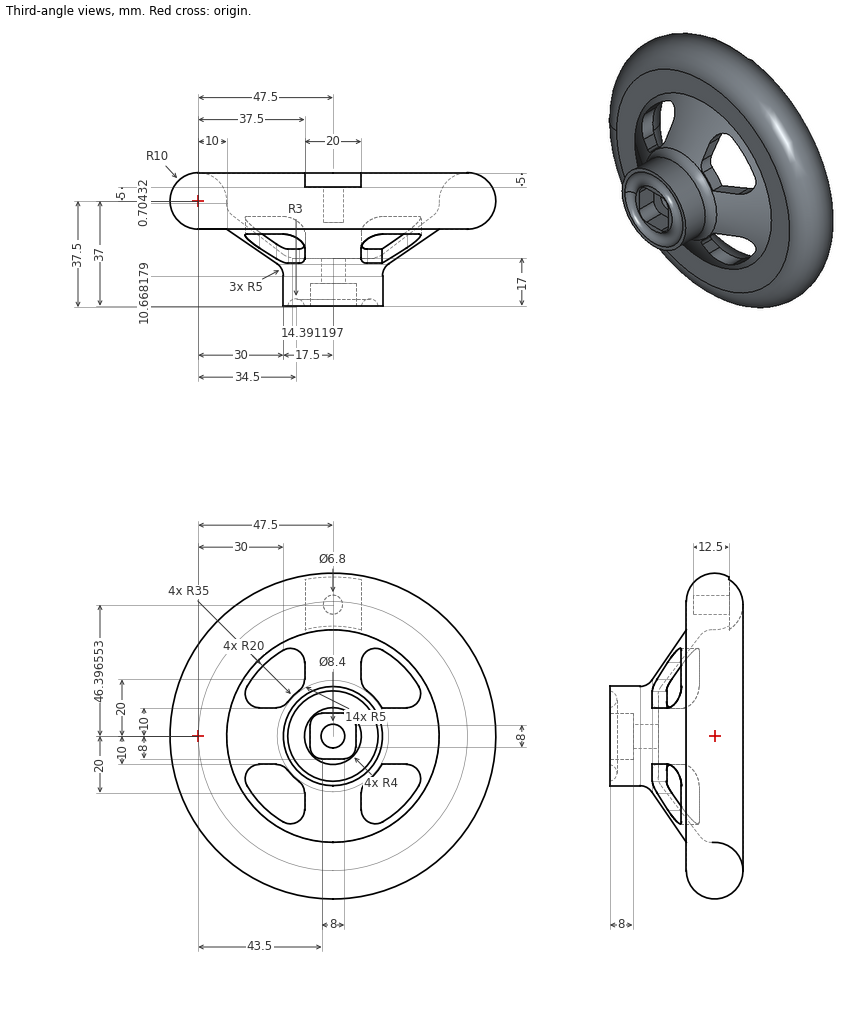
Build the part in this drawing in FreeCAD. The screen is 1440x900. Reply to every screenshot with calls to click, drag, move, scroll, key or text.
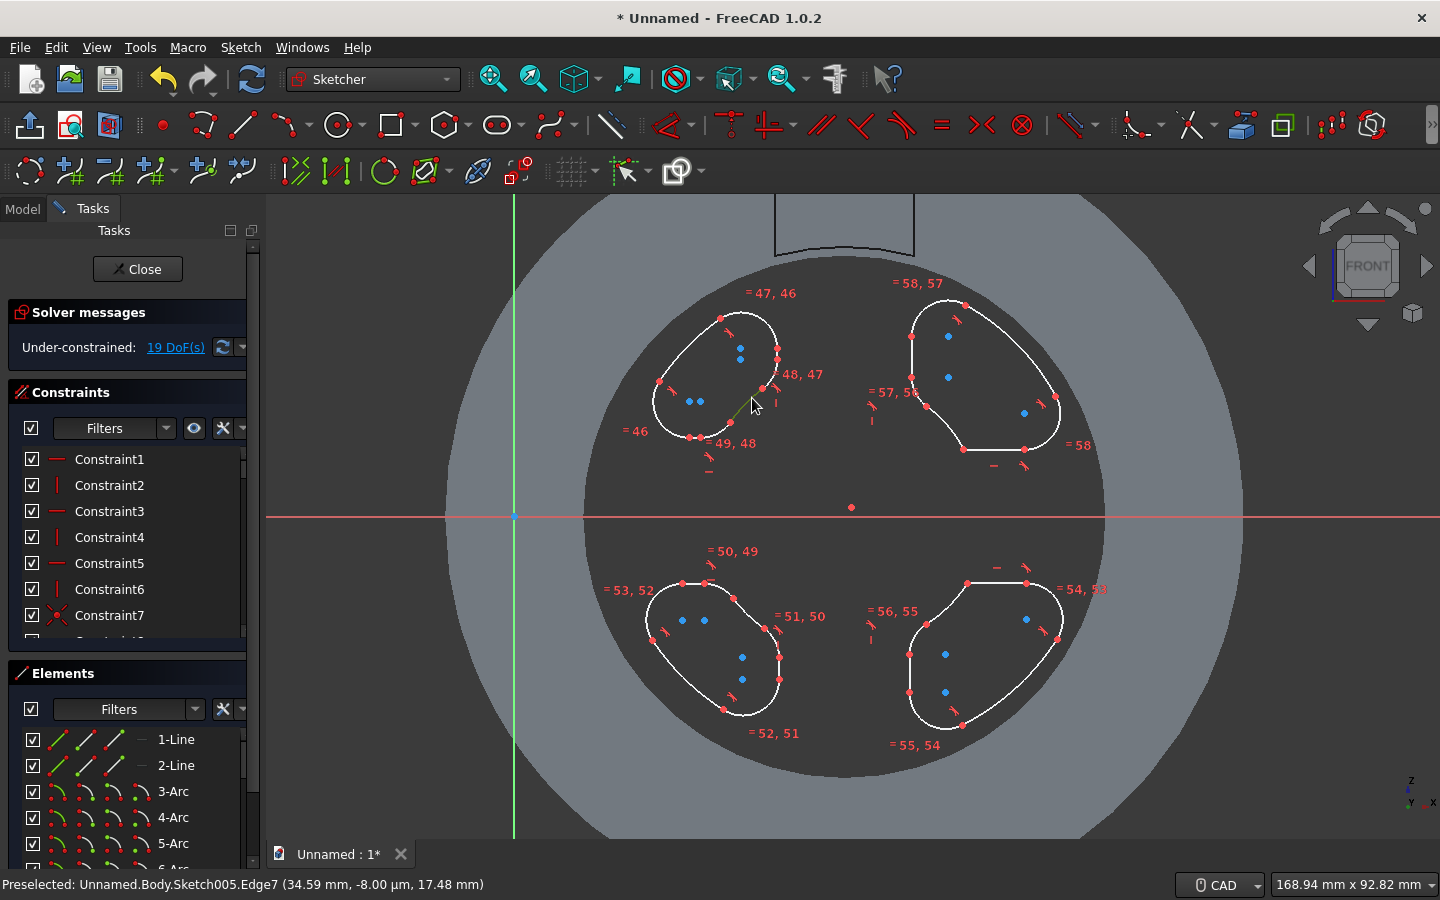
click(741, 608)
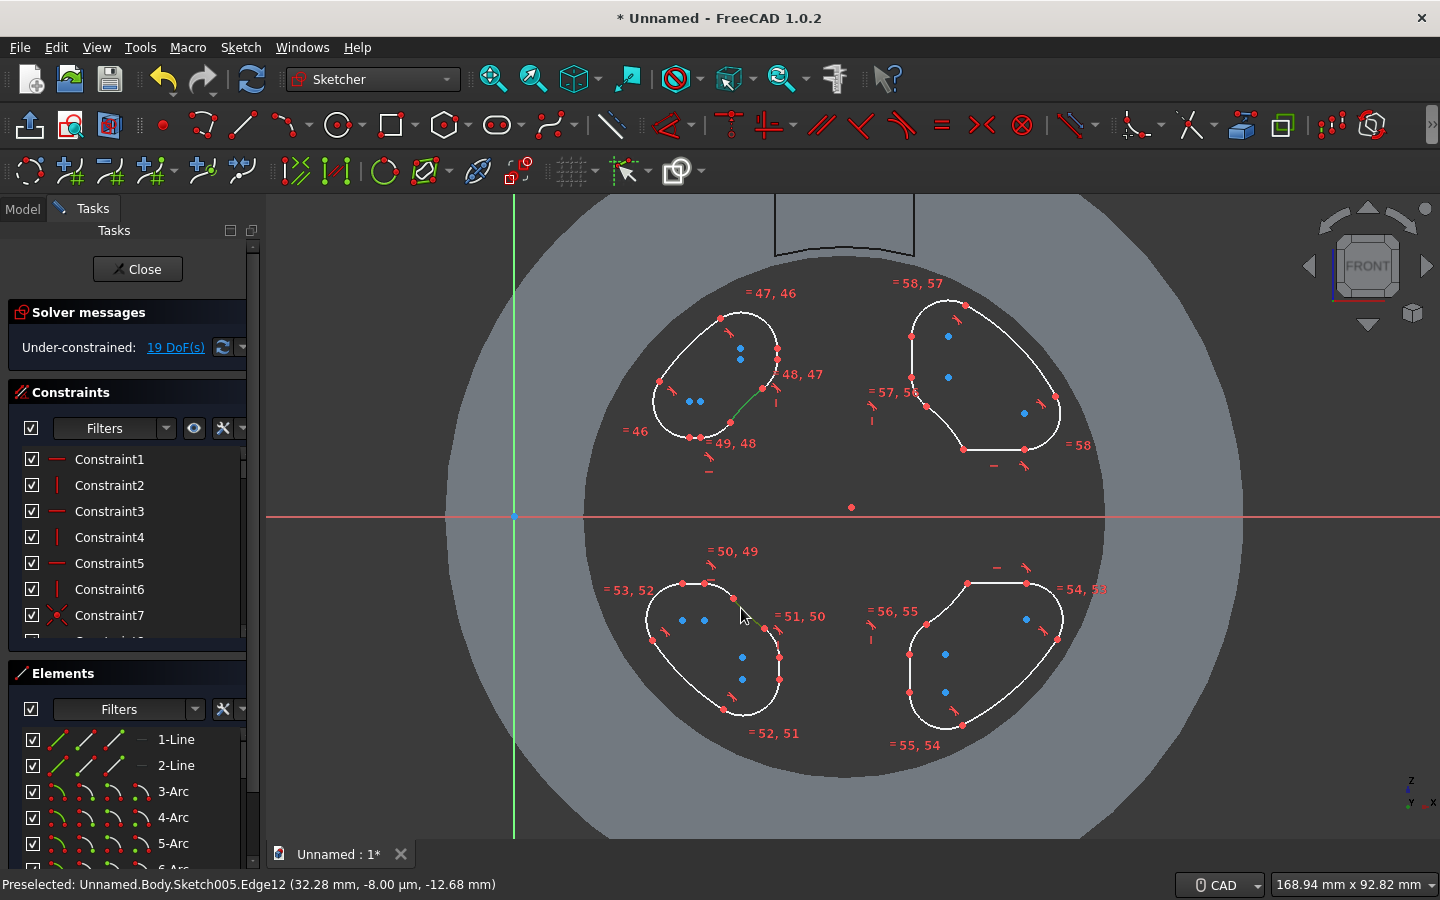
click(940, 614)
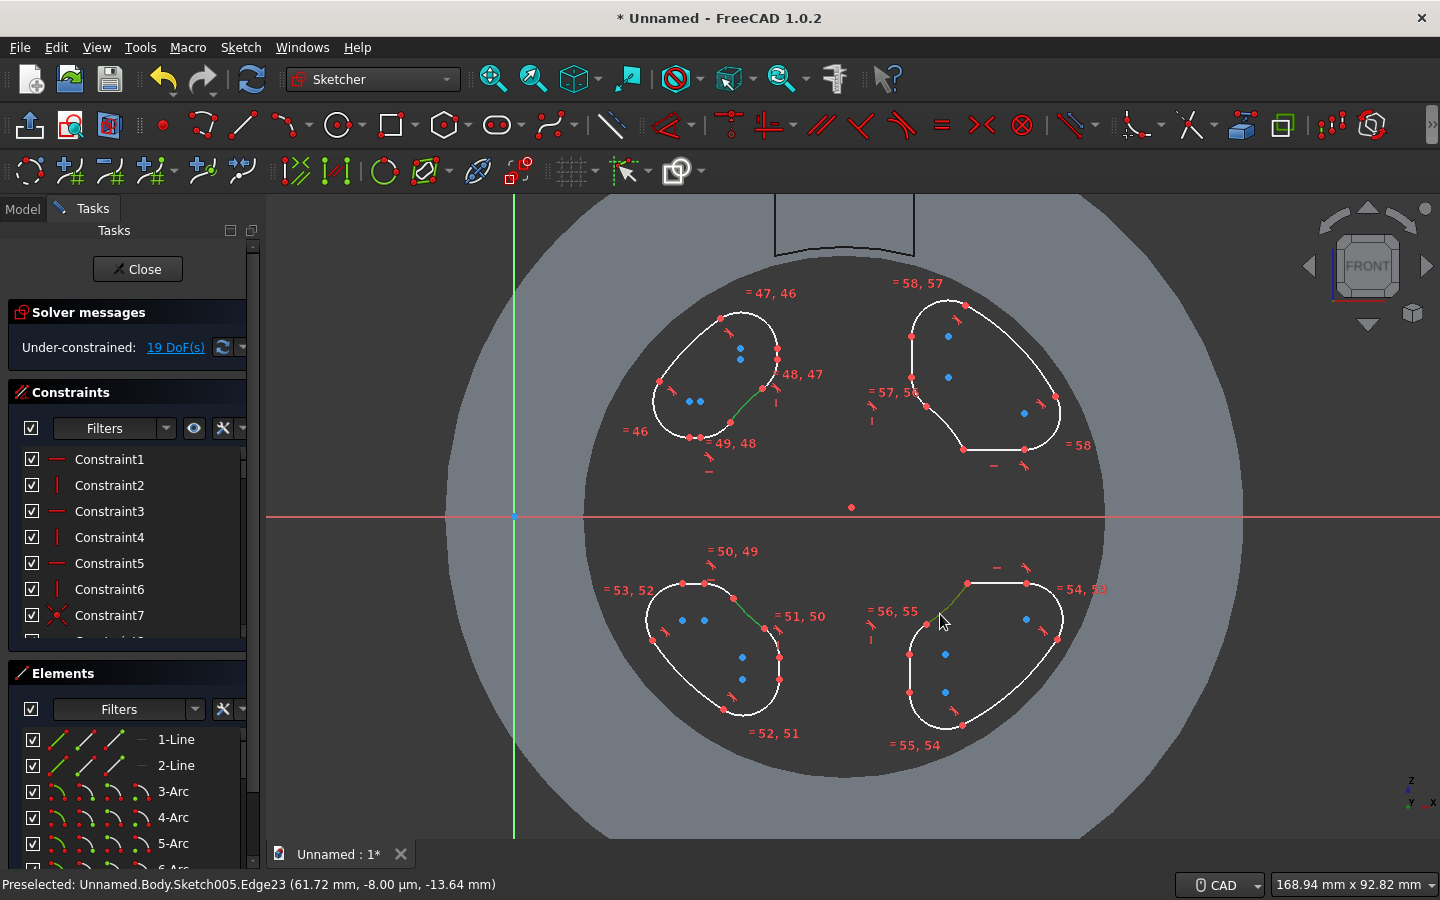
click(955, 435)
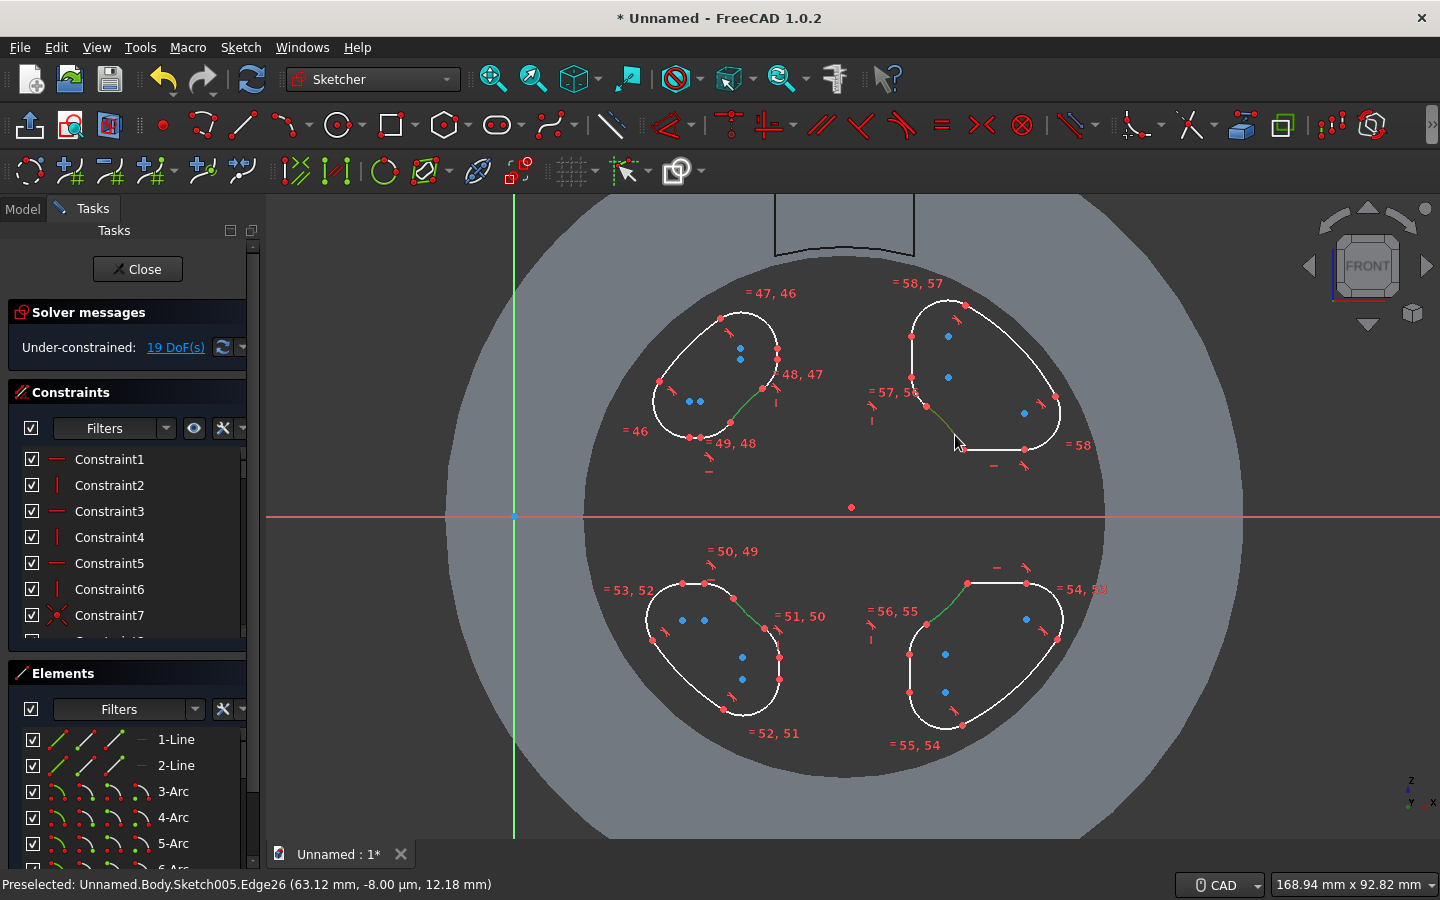
click(942, 126)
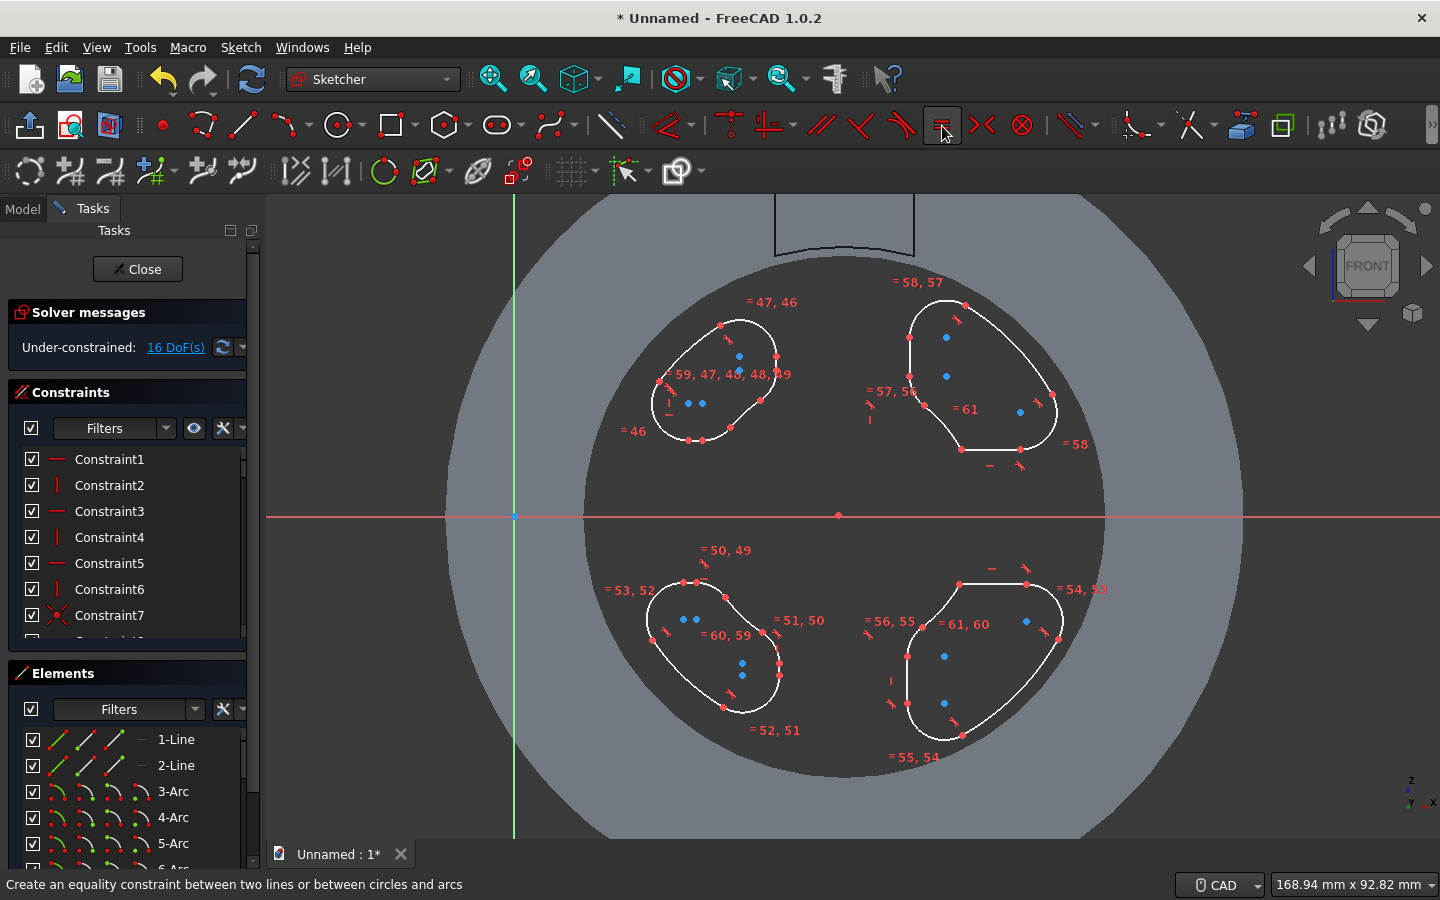
click(700, 340)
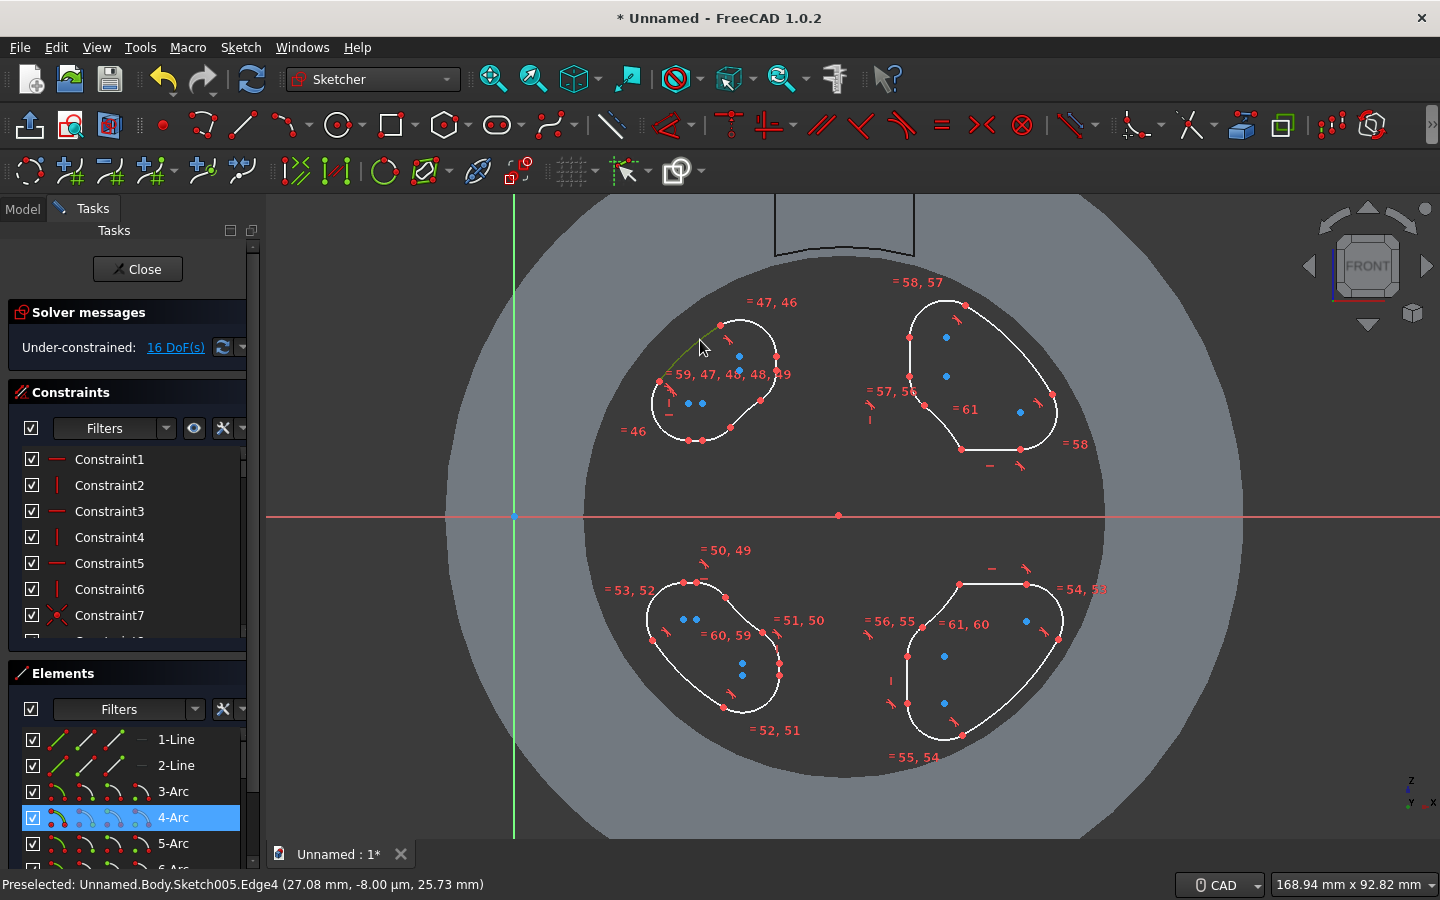
click(671, 663)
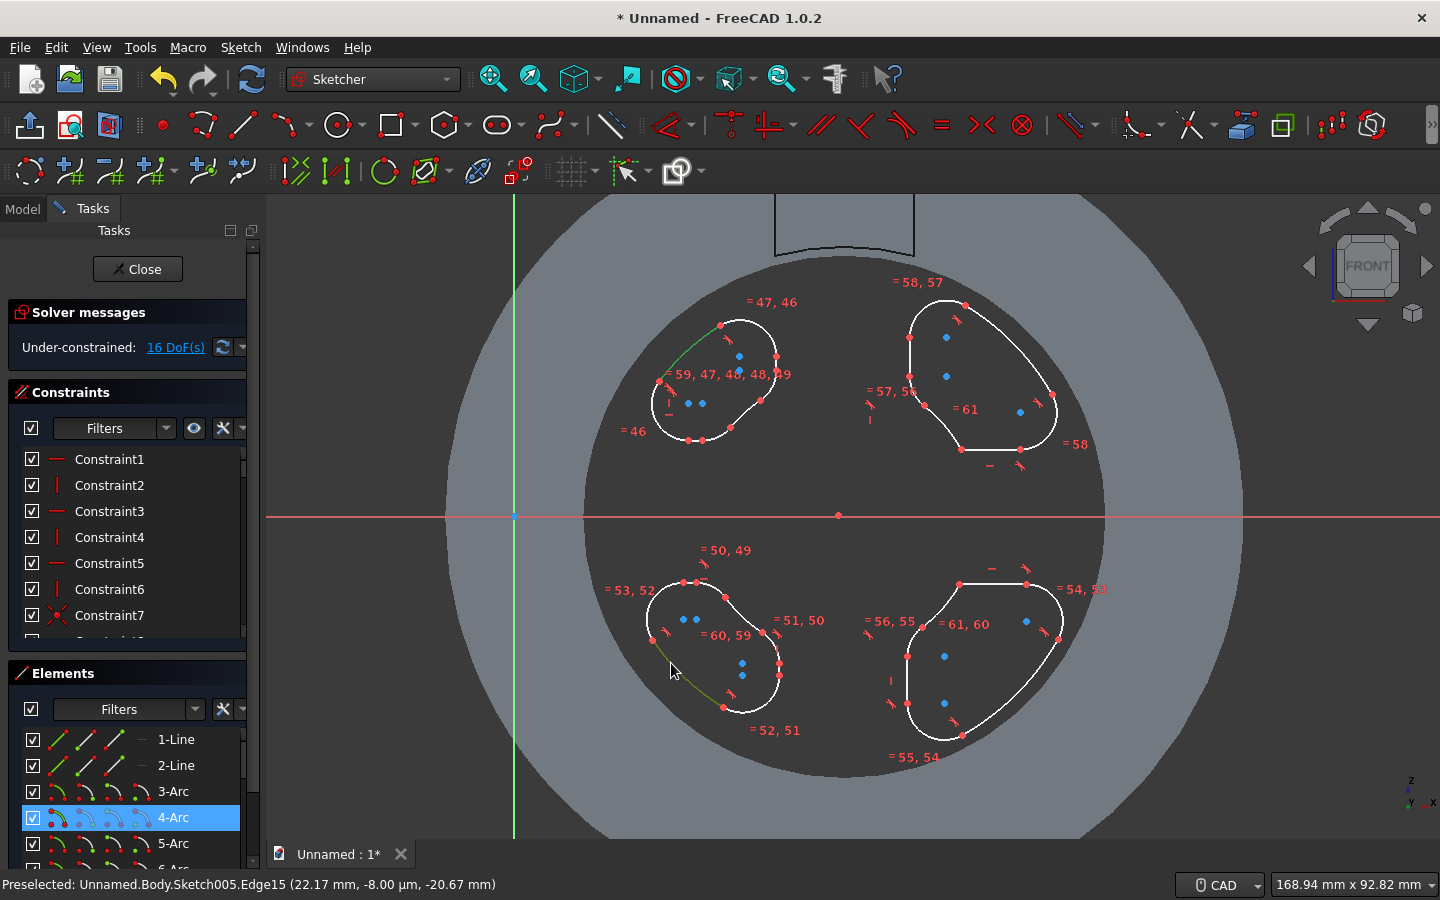
click(996, 712)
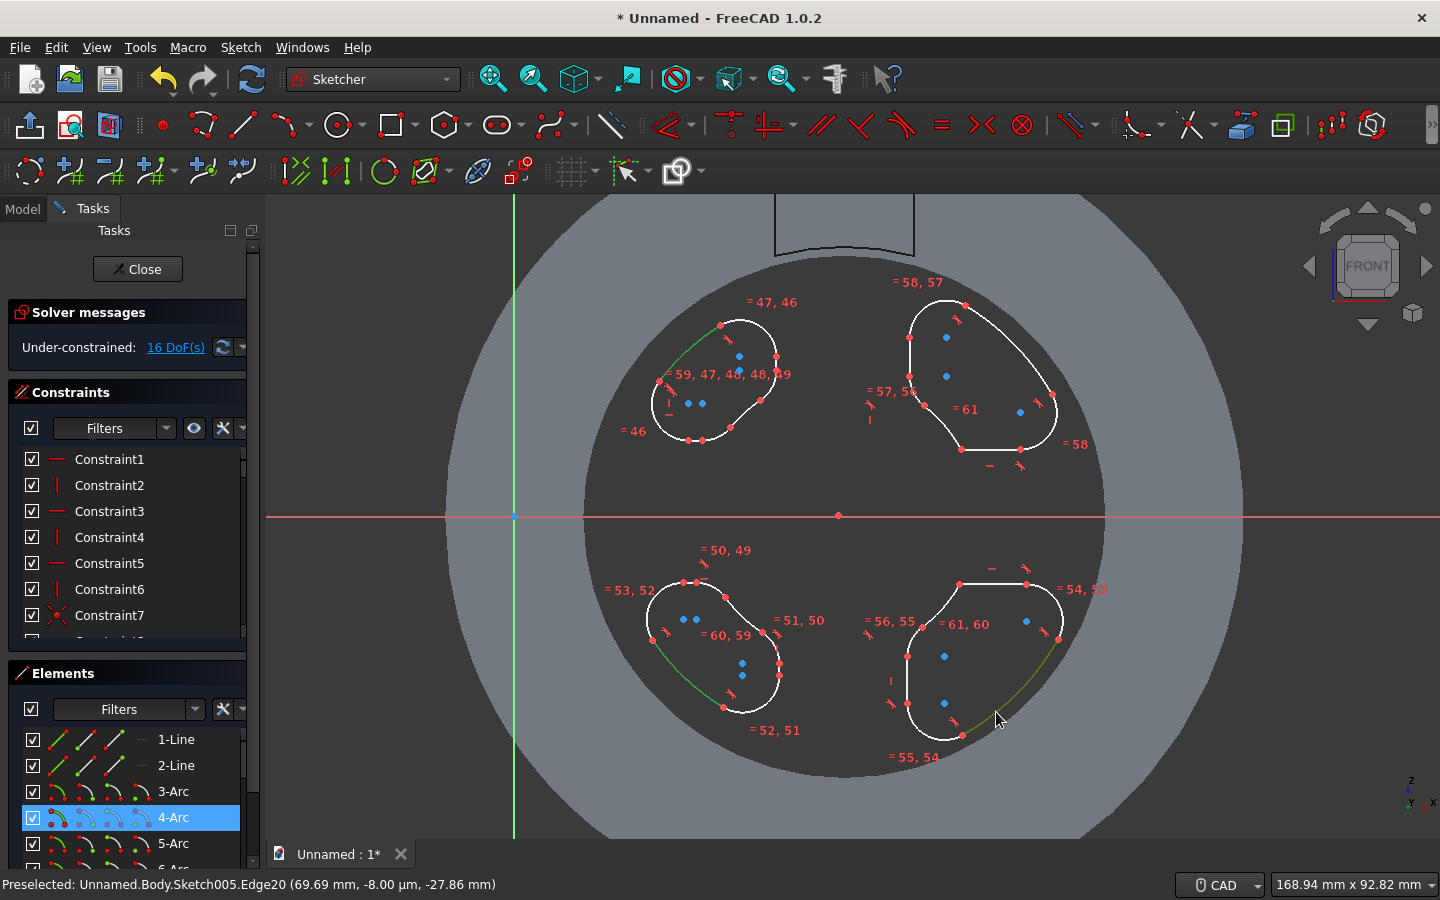
click(1031, 364)